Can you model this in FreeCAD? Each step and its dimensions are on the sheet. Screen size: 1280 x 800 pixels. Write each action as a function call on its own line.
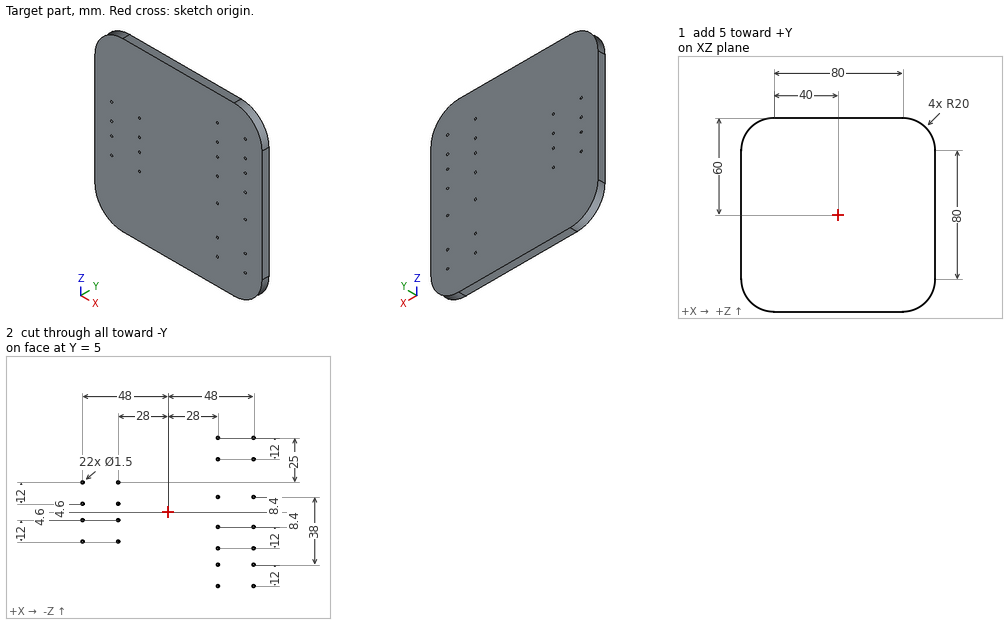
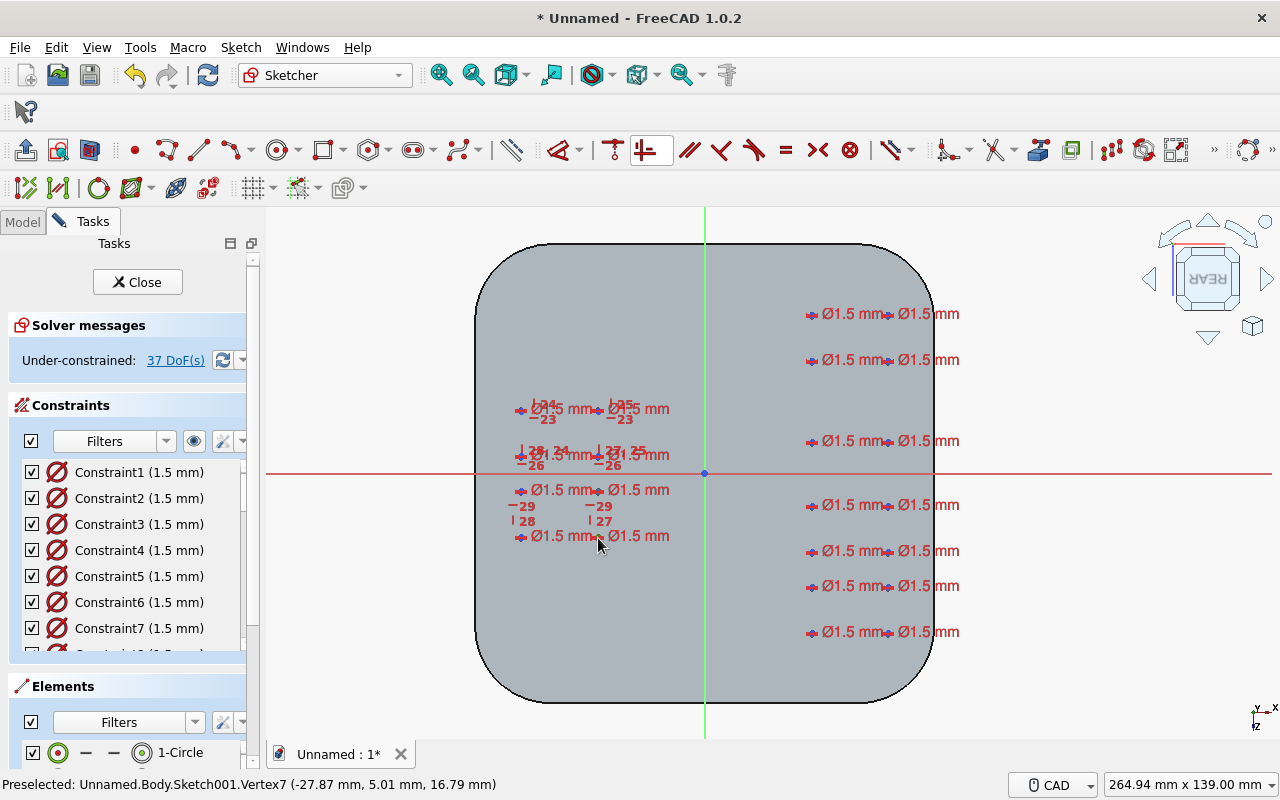
click(668, 150)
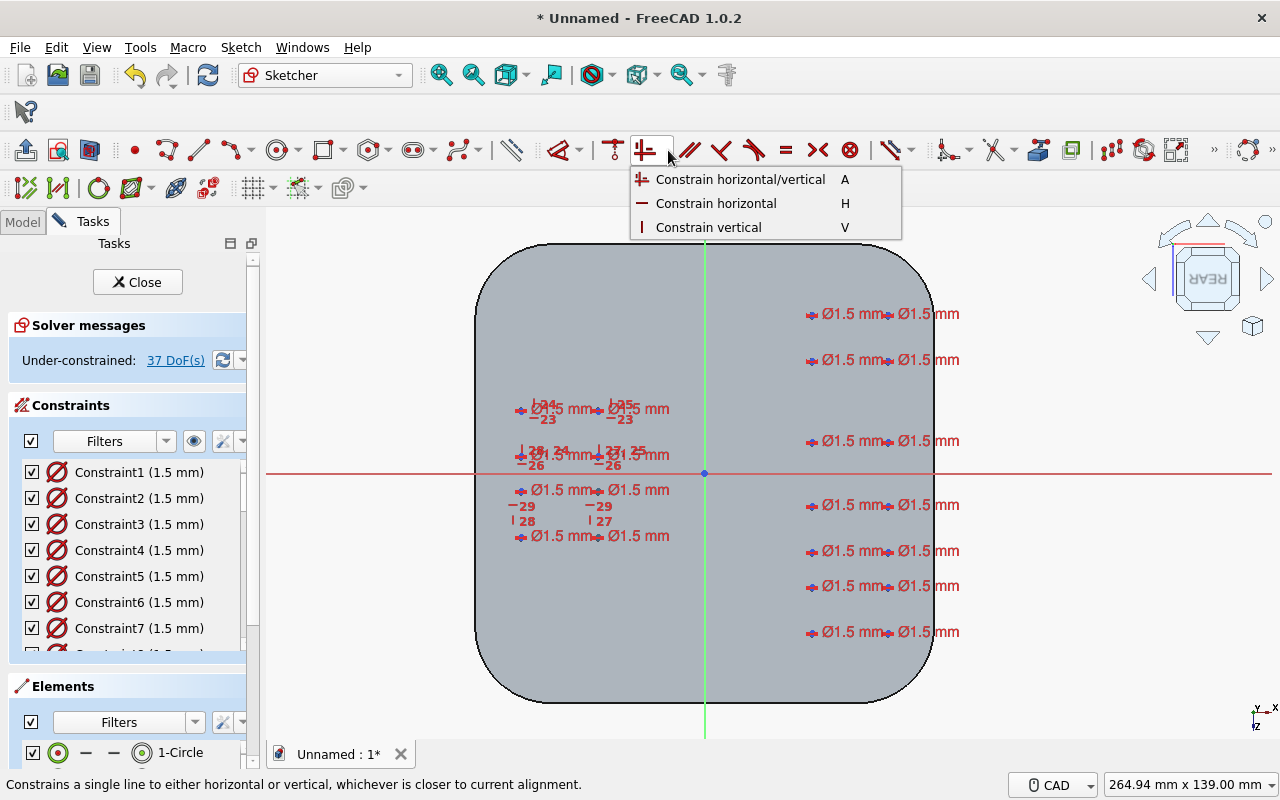
click(766, 227)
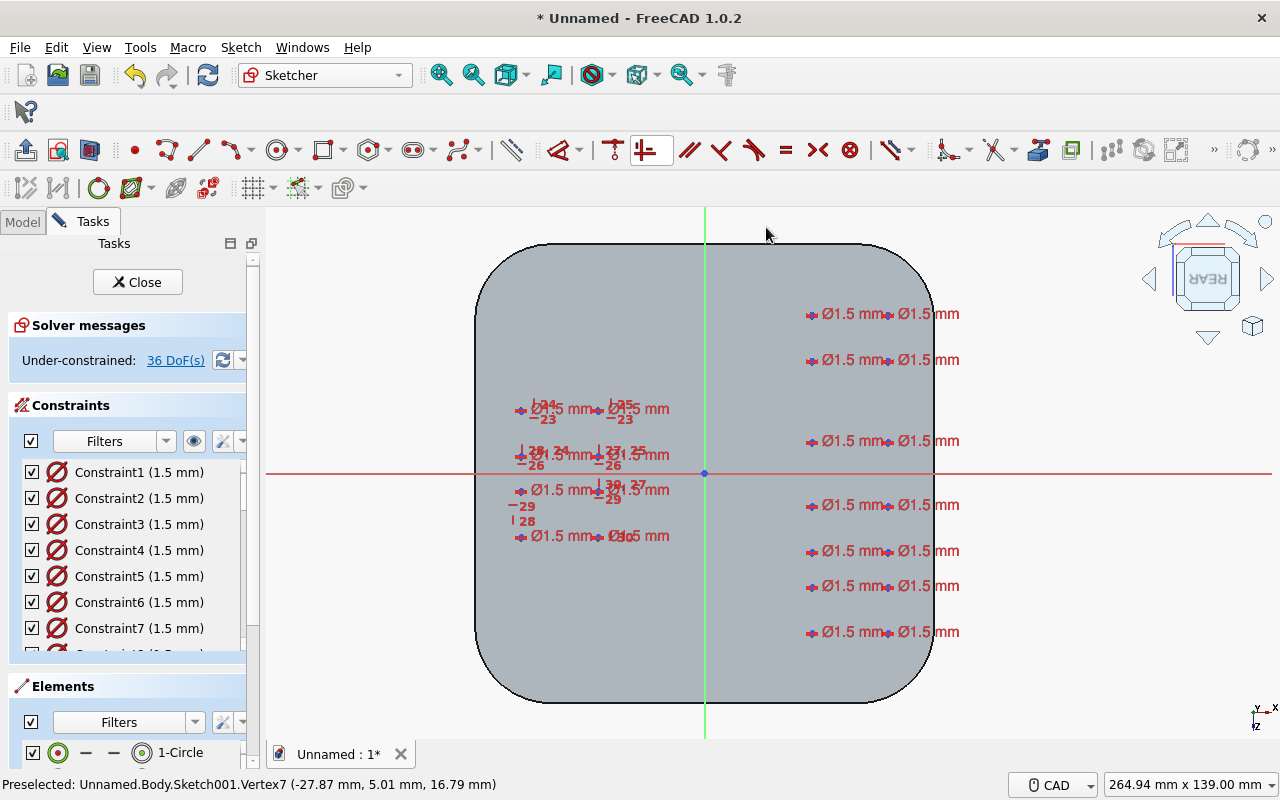
click(521, 492)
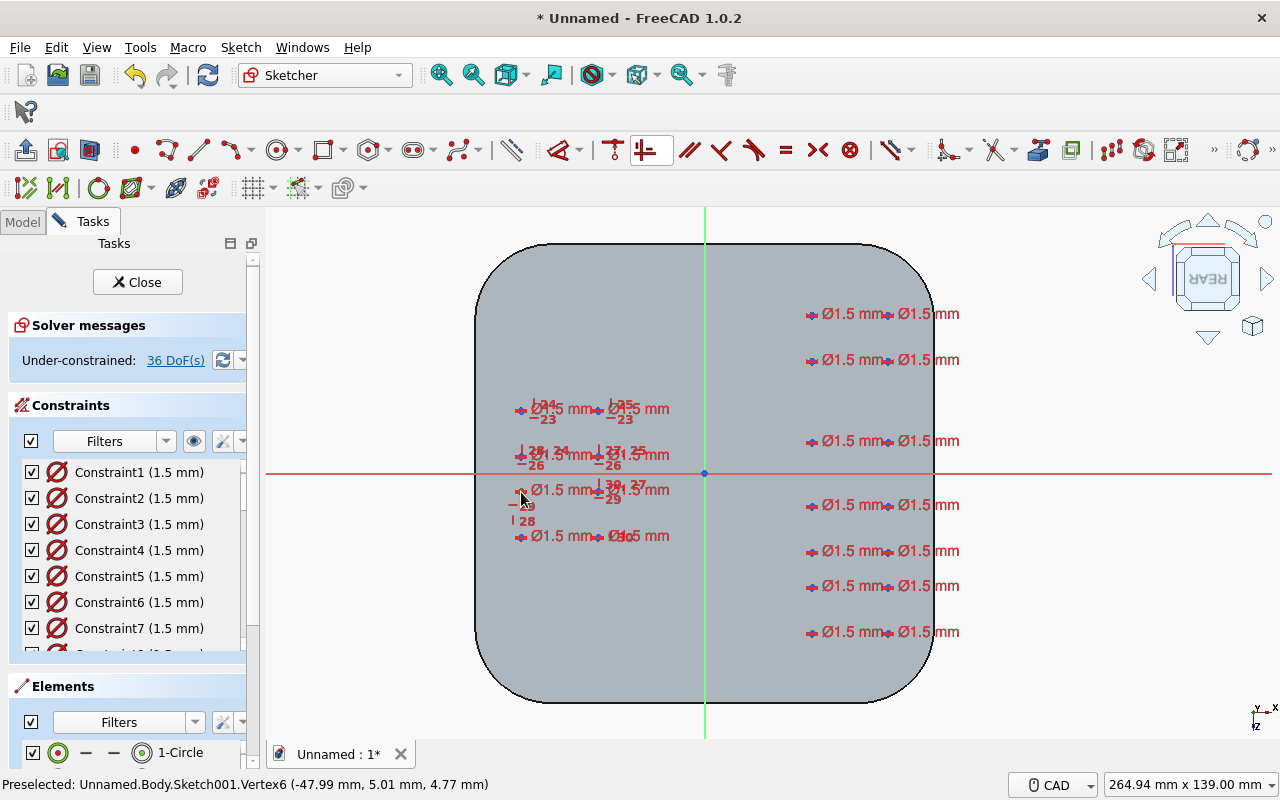
click(521, 538)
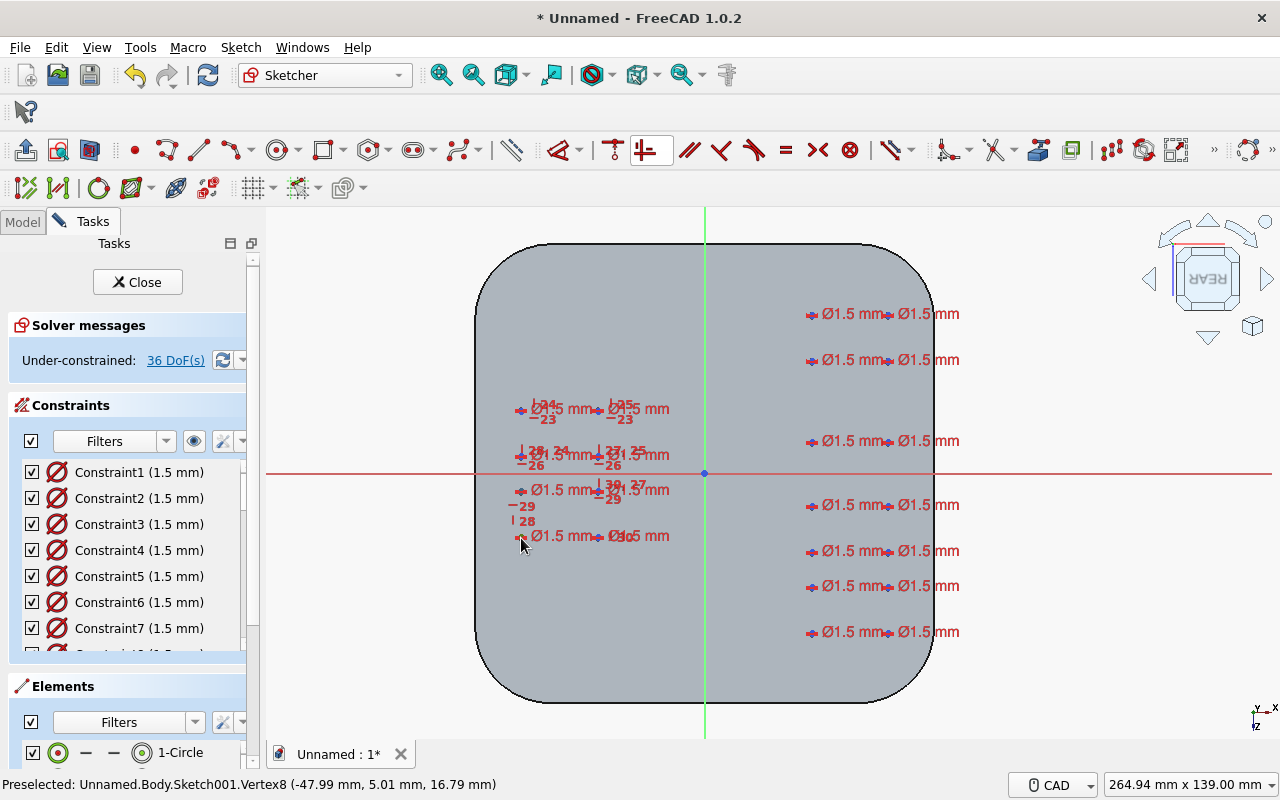
click(668, 150)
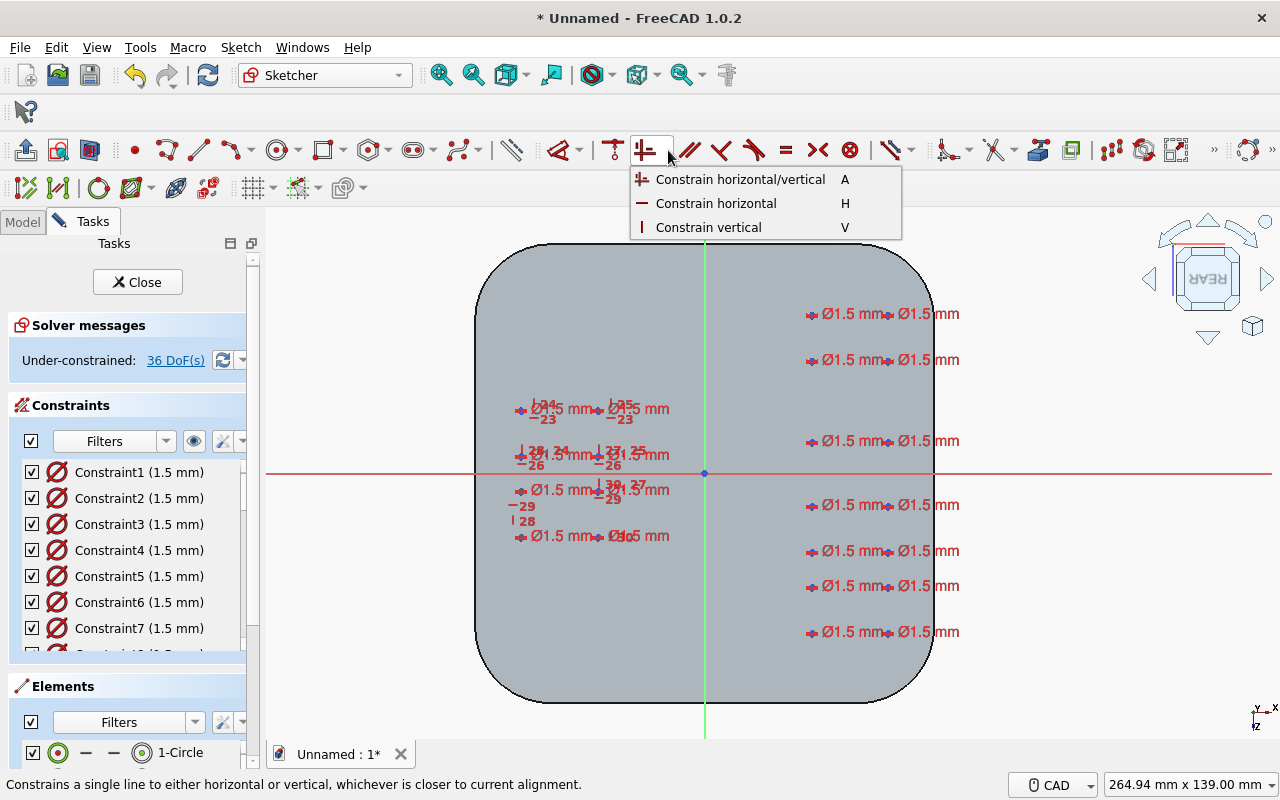
click(766, 227)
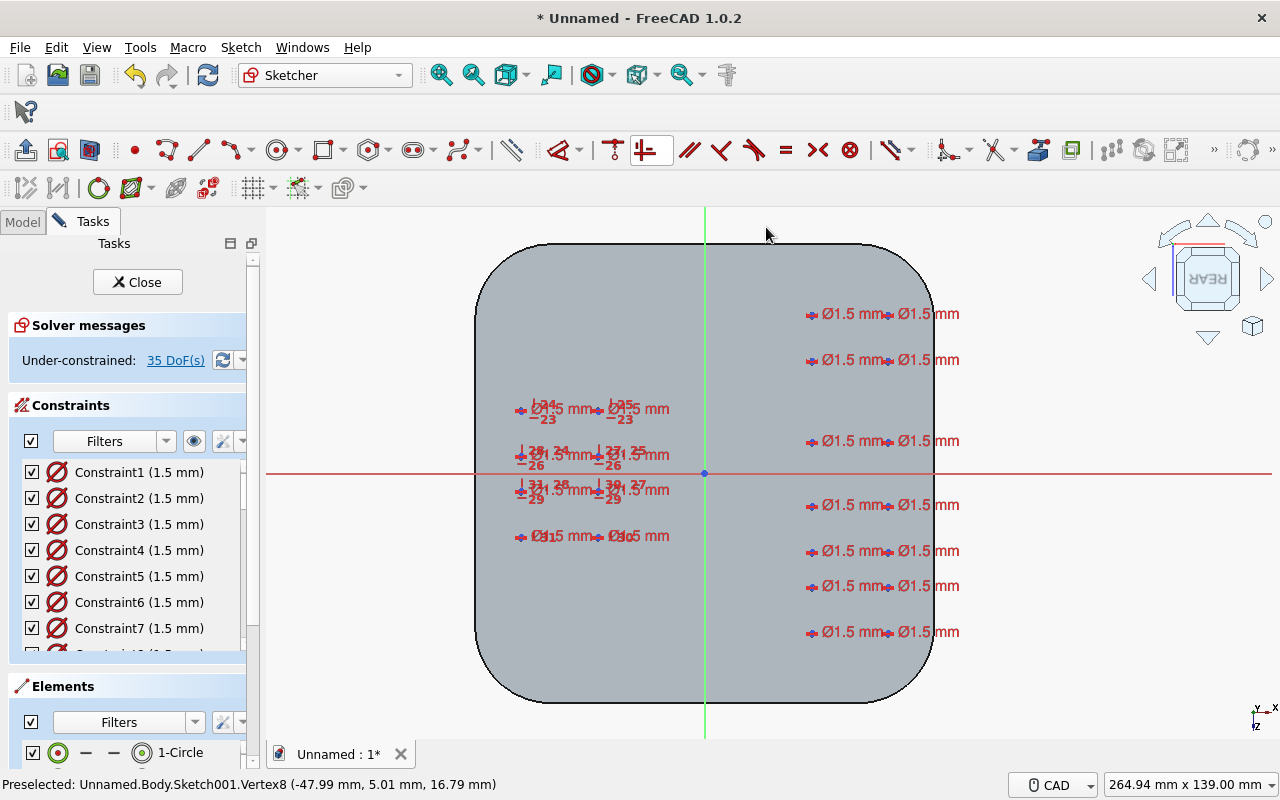
click(598, 538)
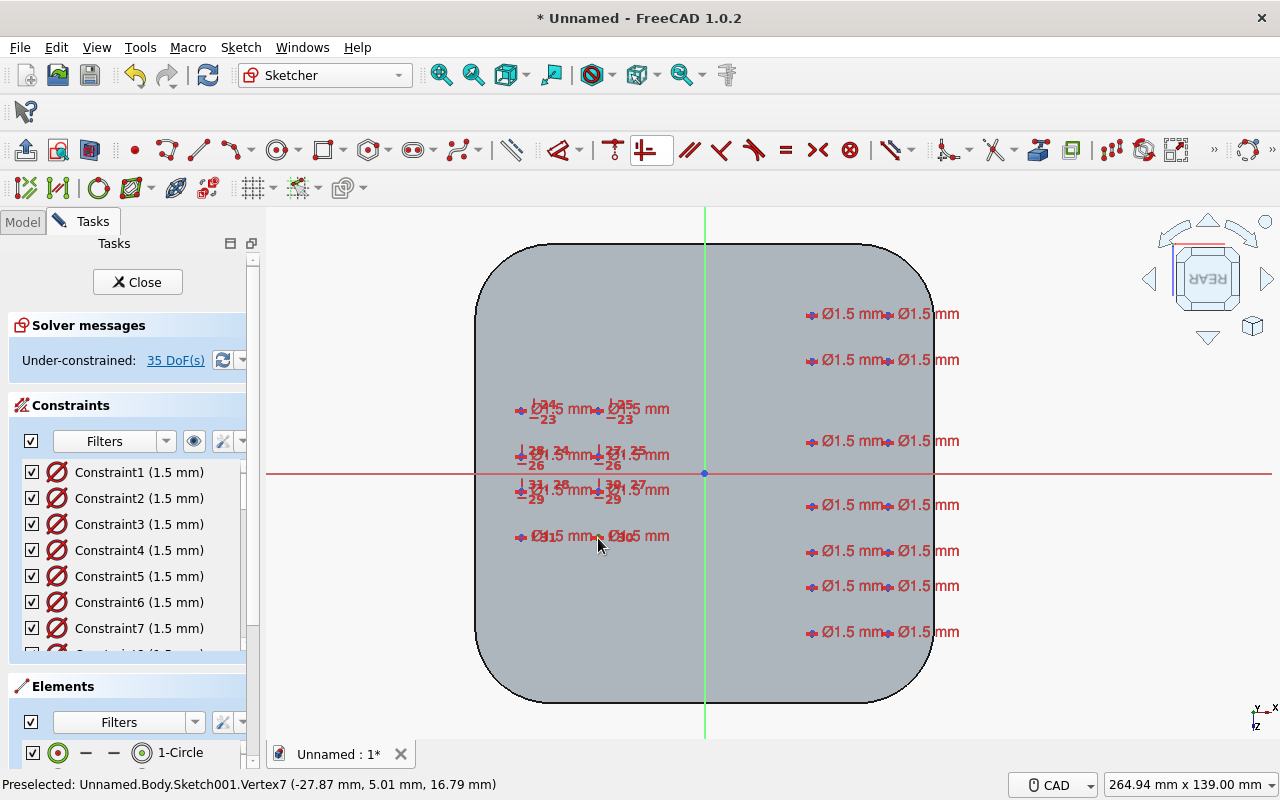
click(521, 538)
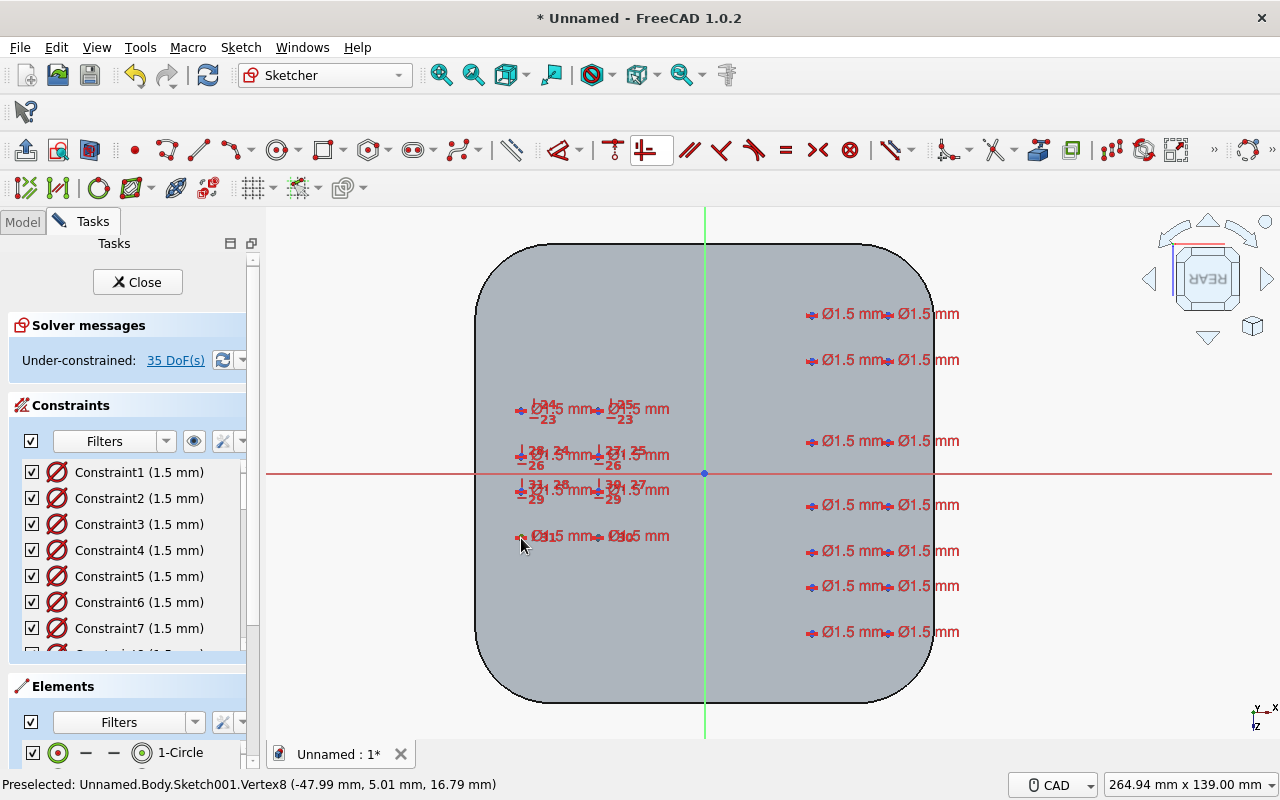
click(668, 150)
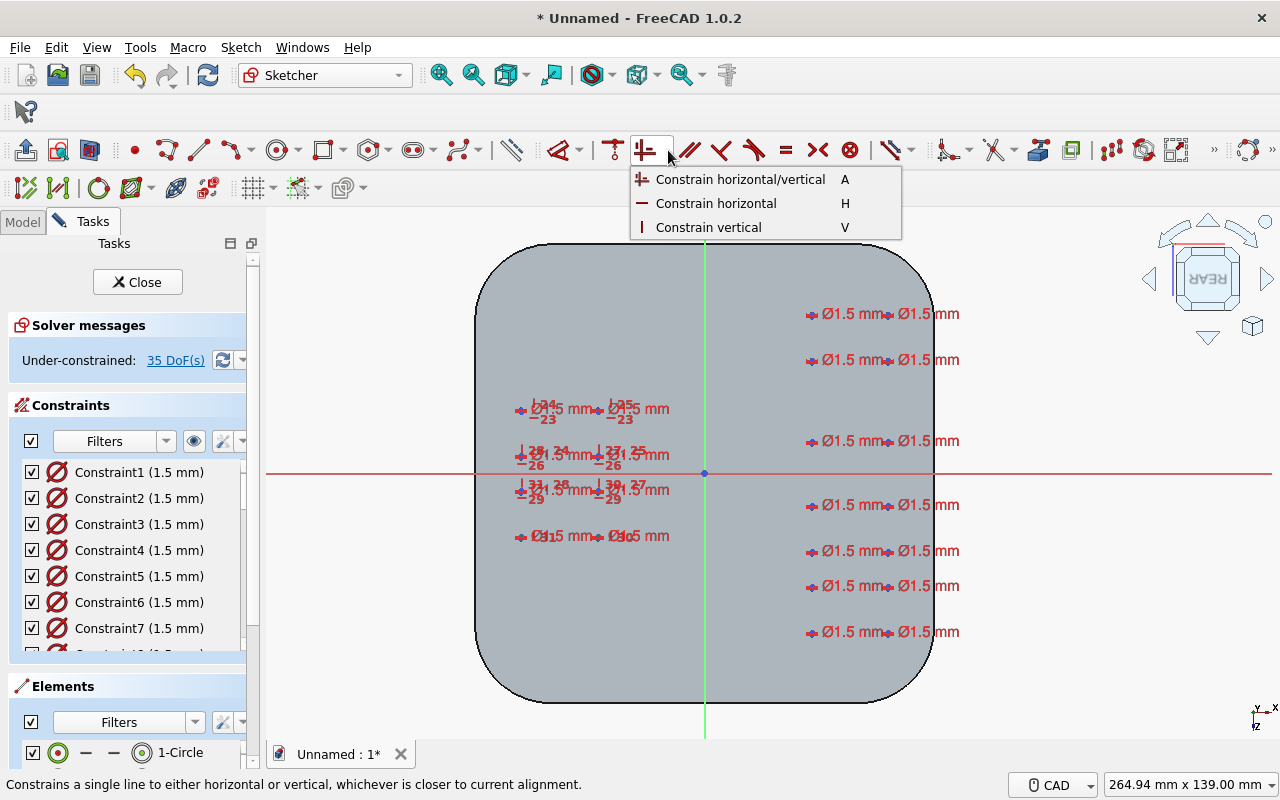
click(766, 203)